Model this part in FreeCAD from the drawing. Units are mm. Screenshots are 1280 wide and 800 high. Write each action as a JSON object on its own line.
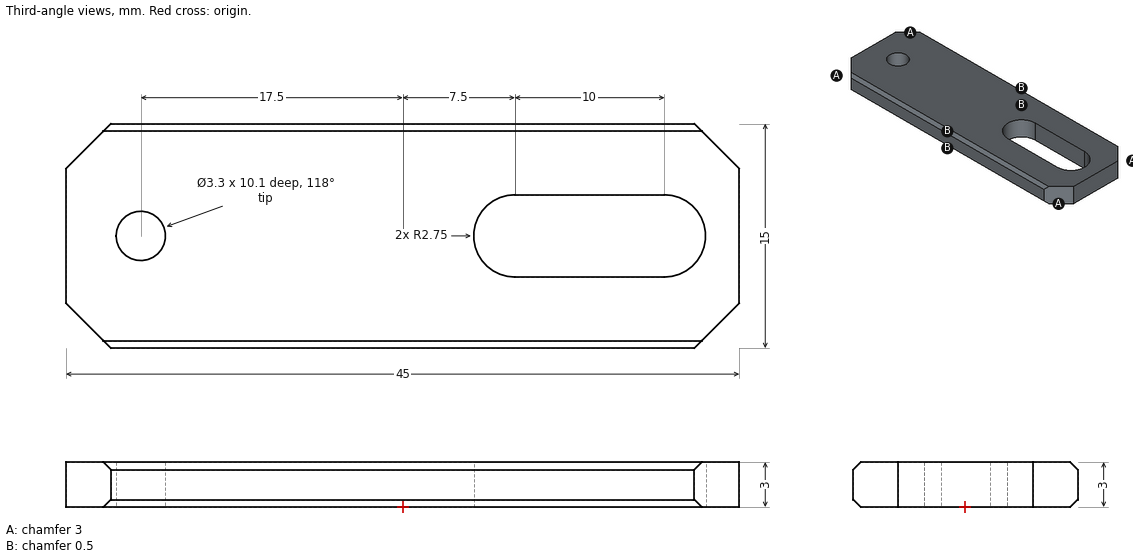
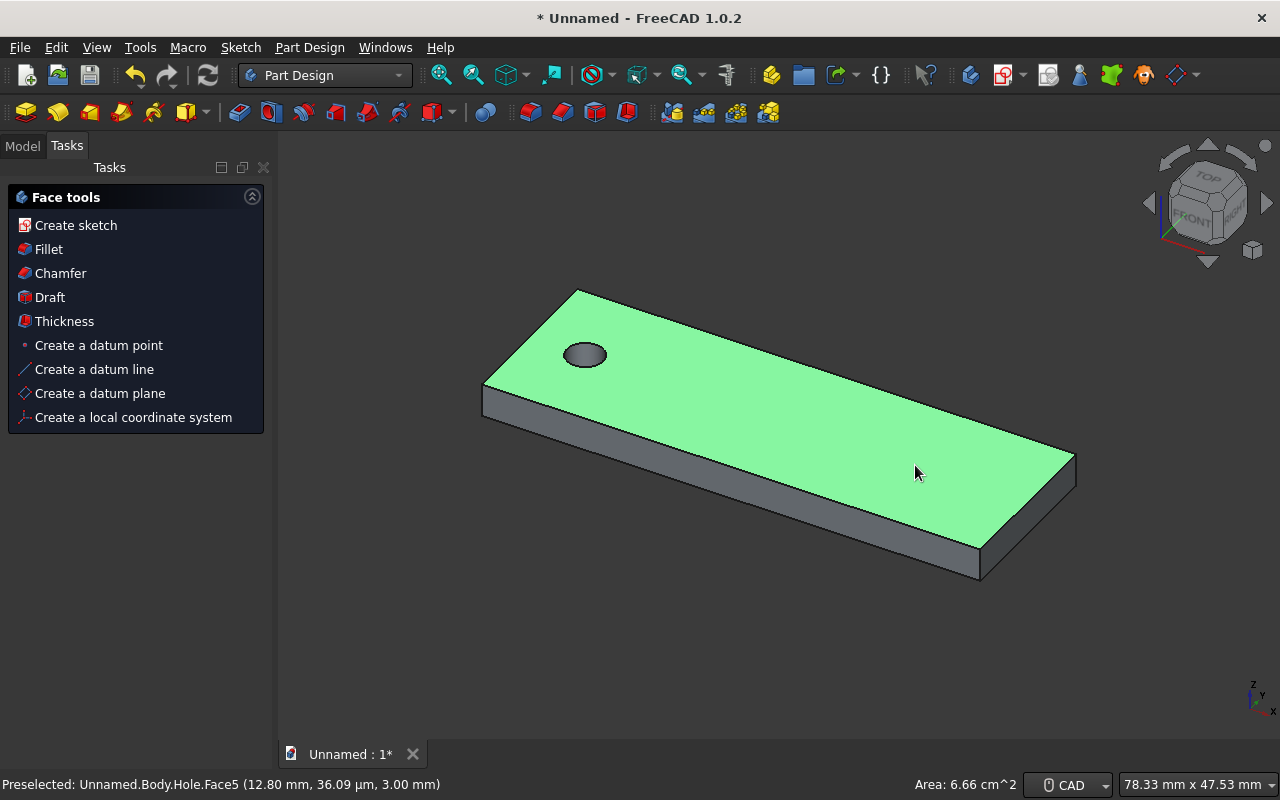
{"action": "left_click", "coordinate": [1004, 76]}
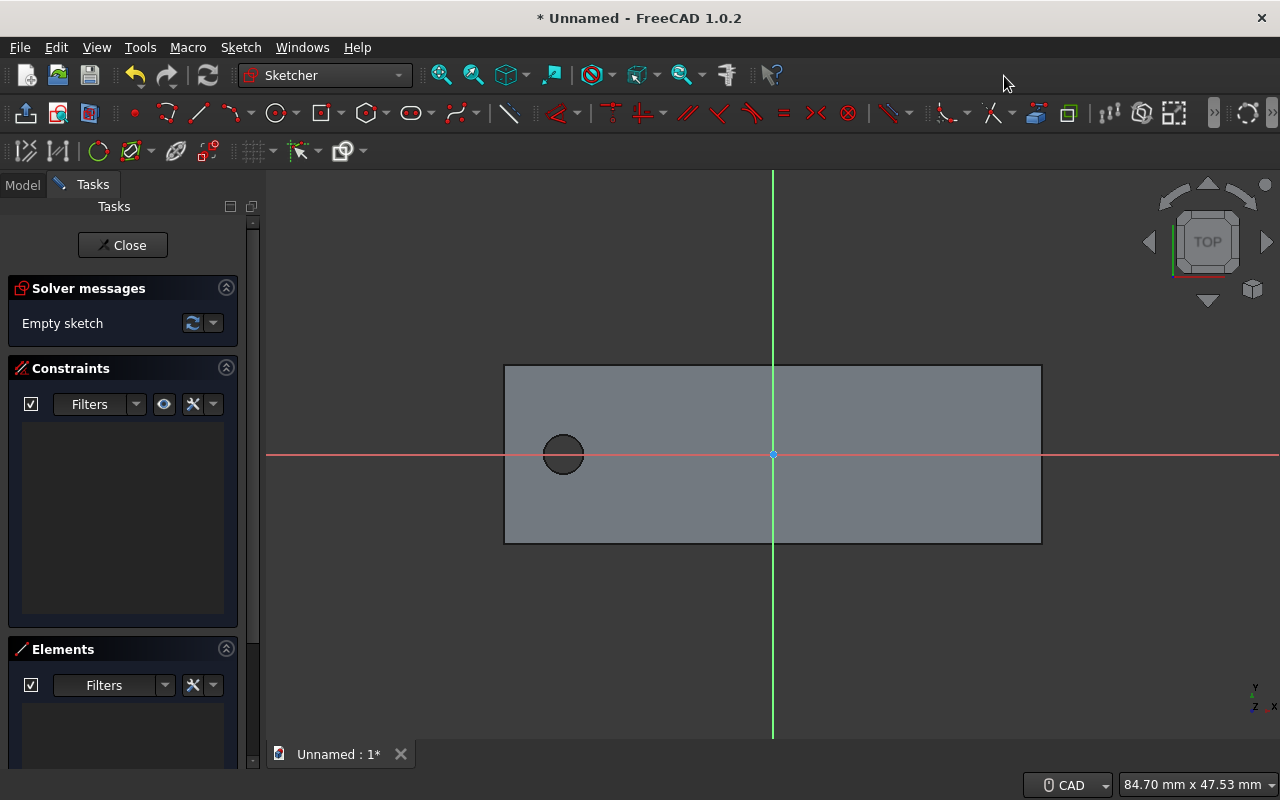
{"action": "scroll", "coordinate": [1049, 455], "scroll_direction": "up", "scroll_amount": 4}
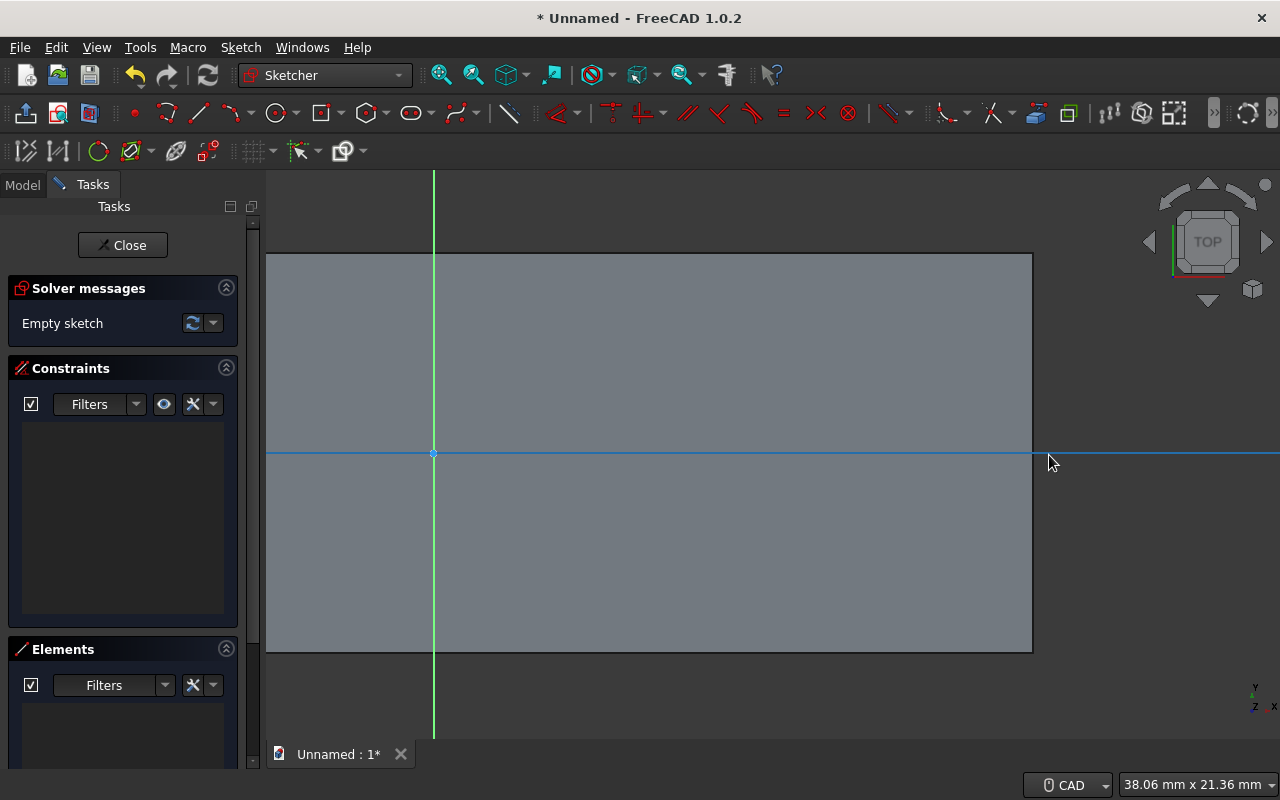
{"action": "left_click", "coordinate": [412, 114]}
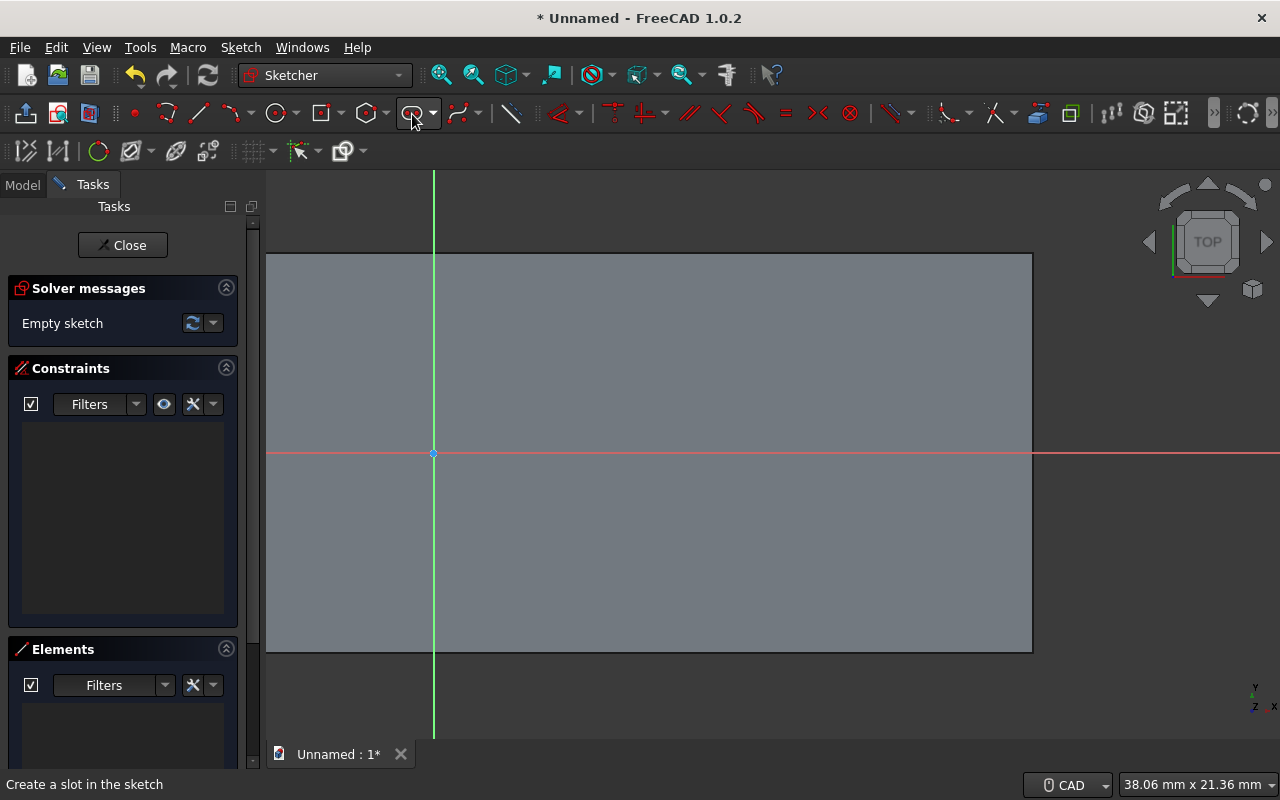
{"action": "left_click", "coordinate": [634, 453]}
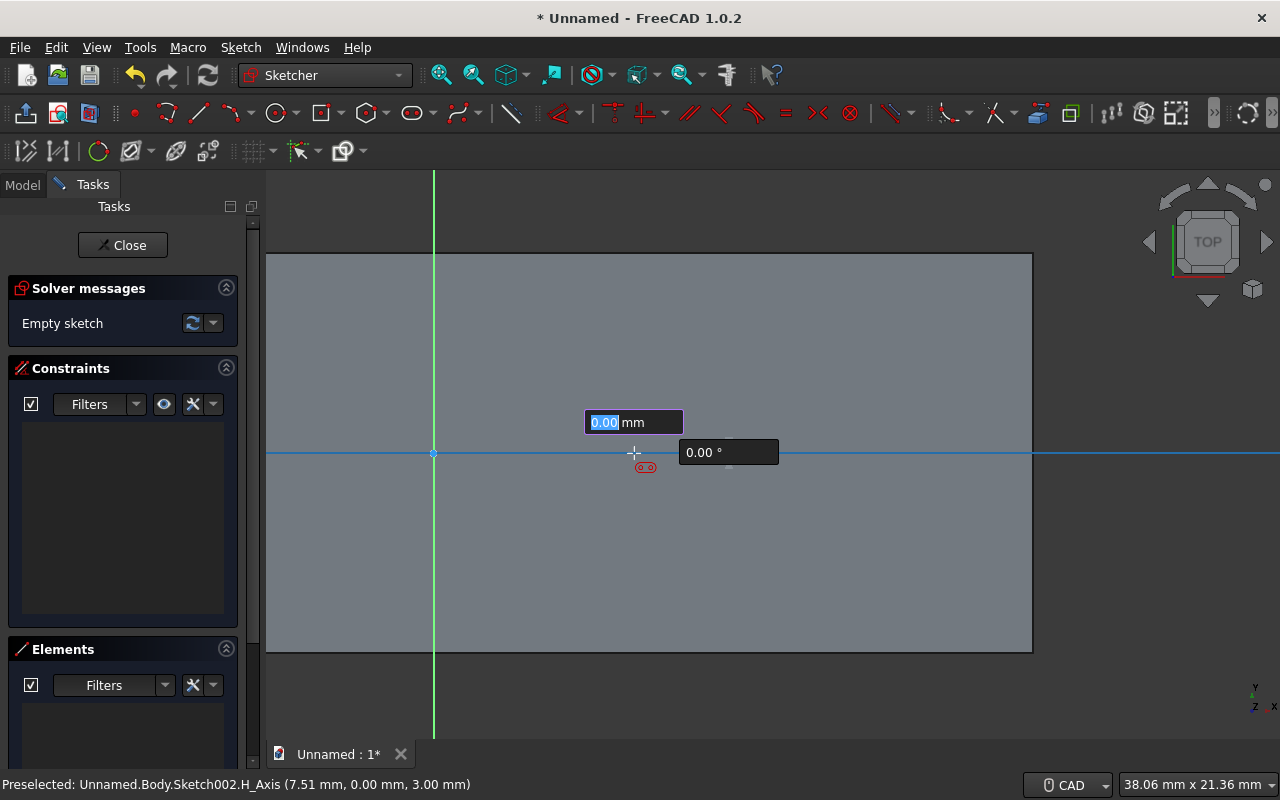
{"action": "left_click", "coordinate": [900, 444]}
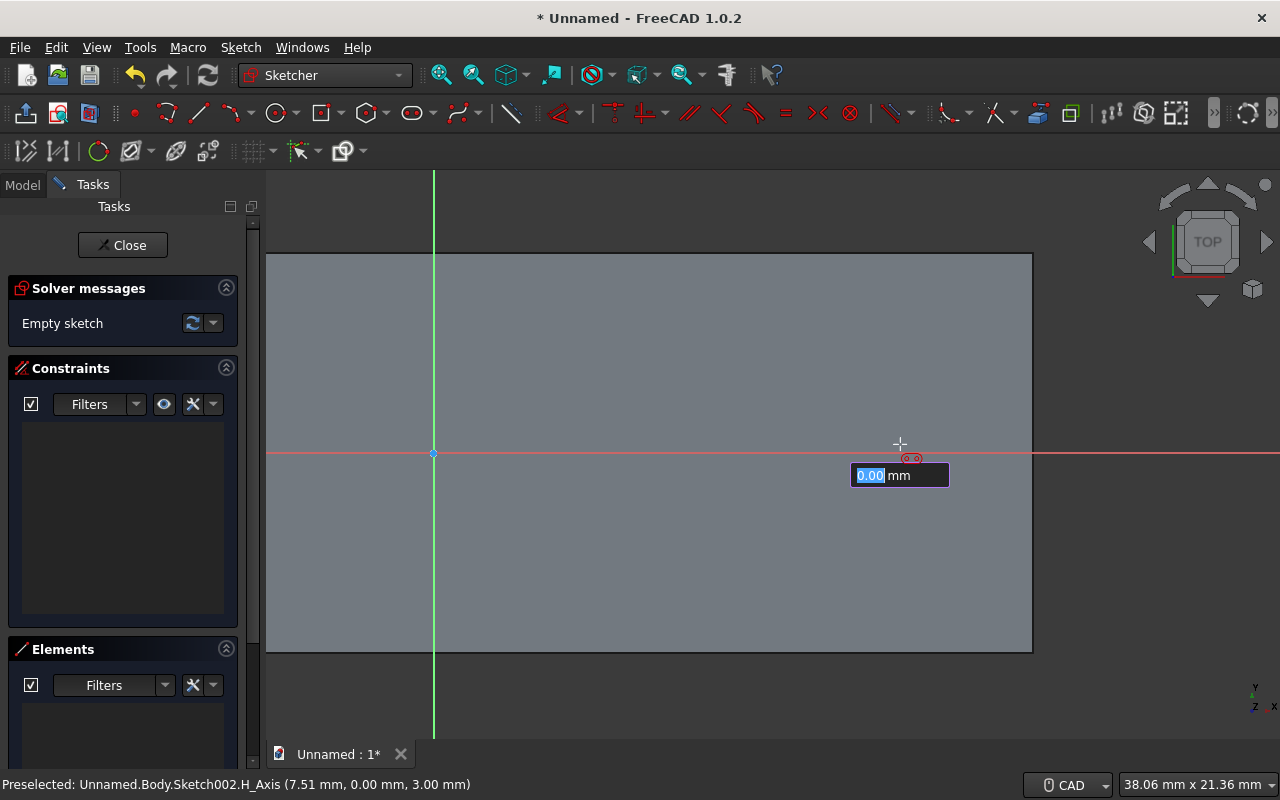
{"action": "left_click", "coordinate": [767, 380]}
{"action": "key", "text": "Escape"}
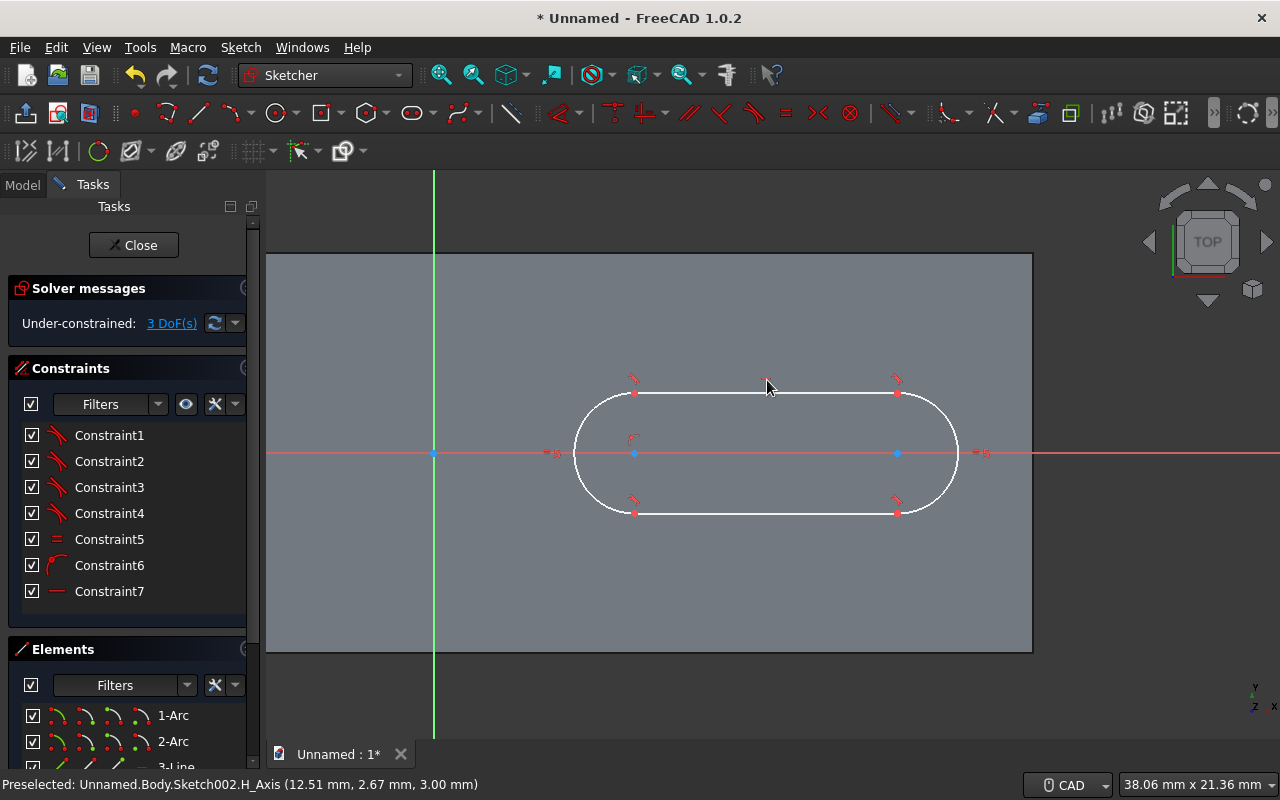
{"action": "left_click", "coordinate": [586, 418]}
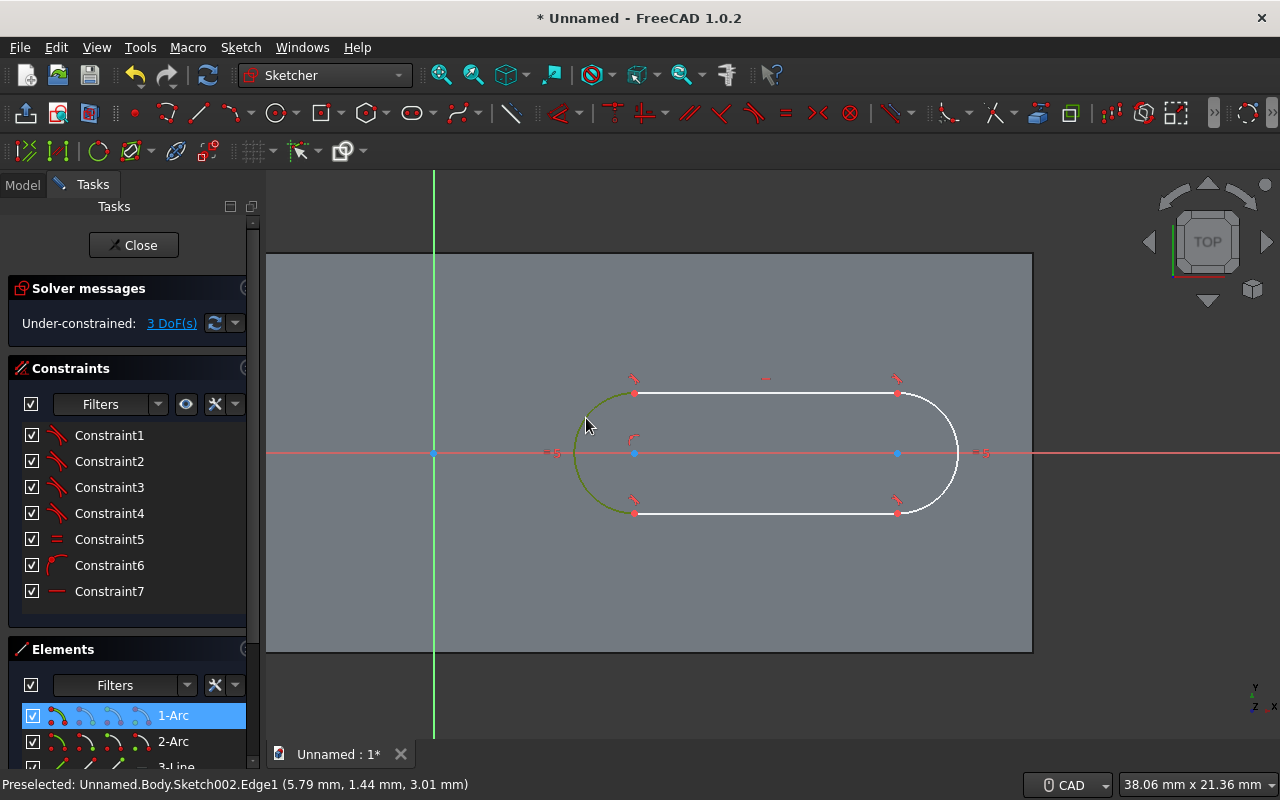
{"action": "left_click", "coordinate": [582, 114]}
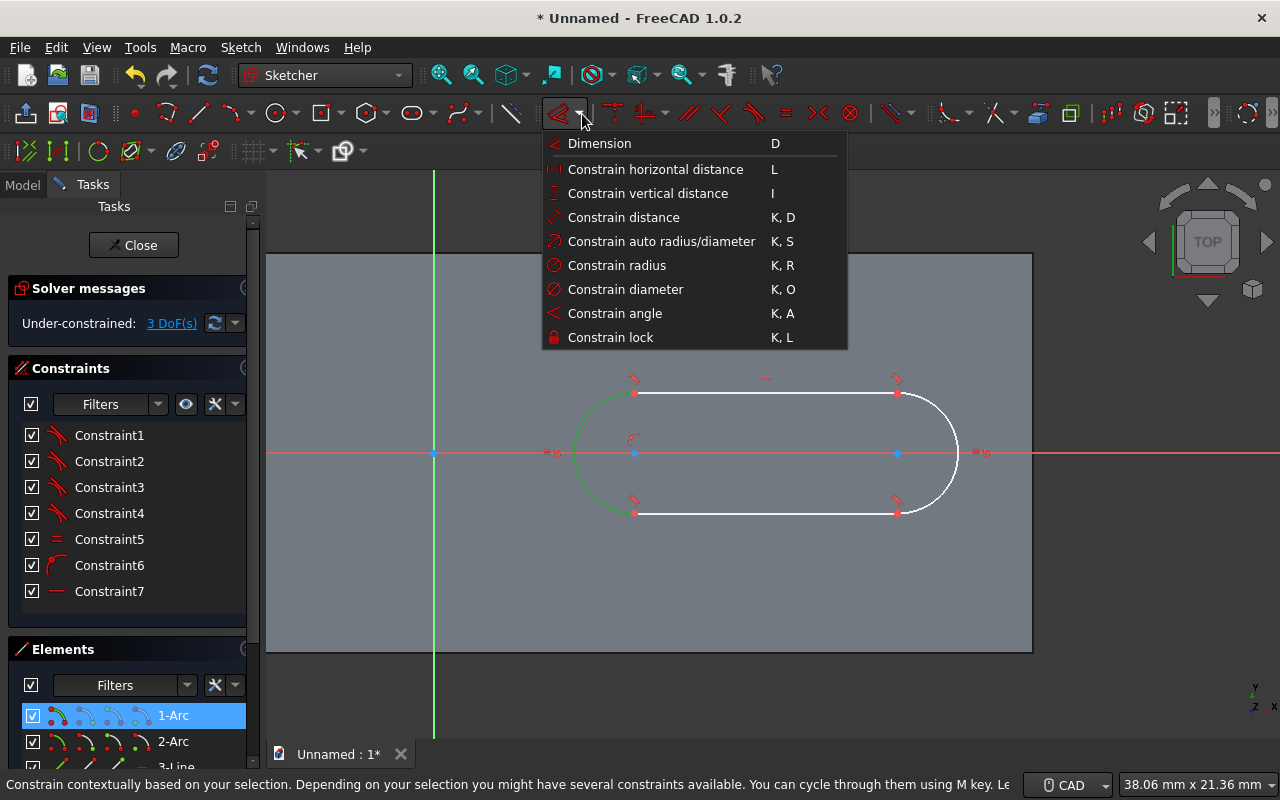
{"action": "left_click", "coordinate": [695, 265]}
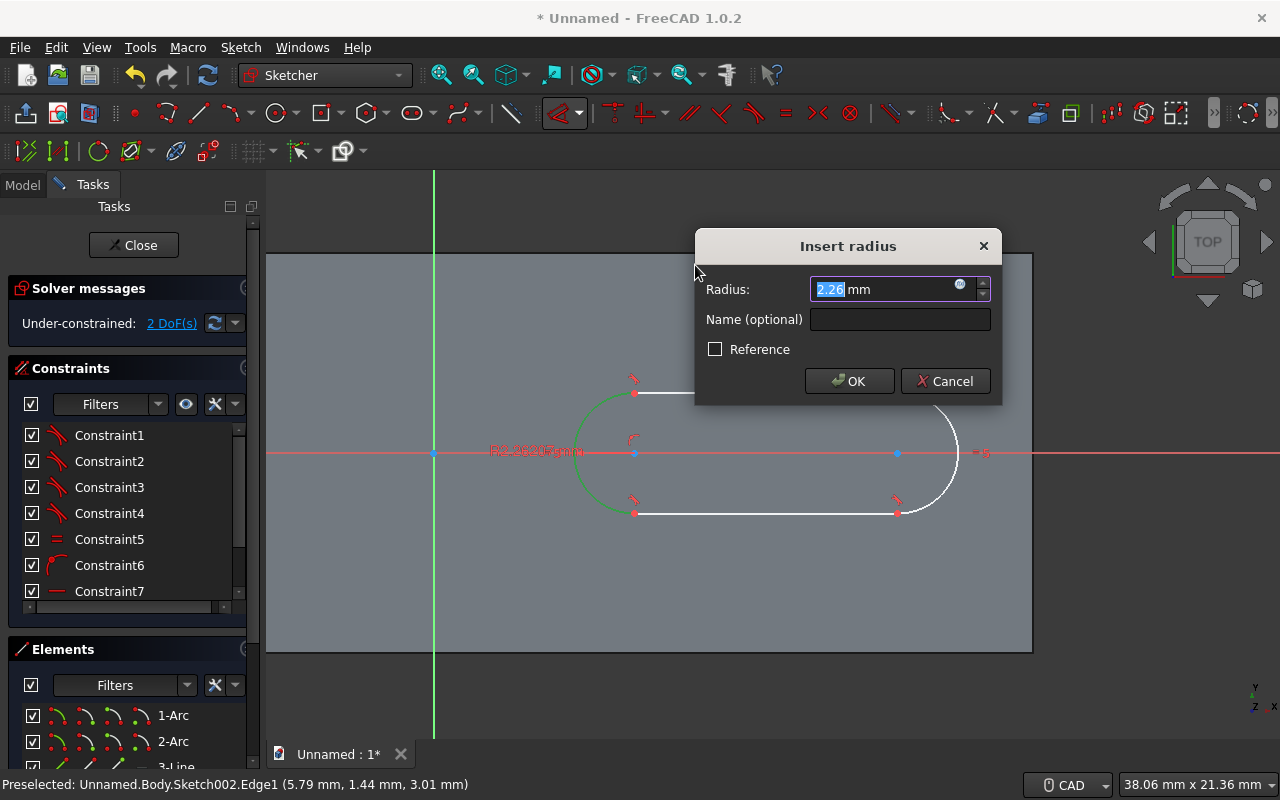
{"action": "type", "text": "2.75"}
{"action": "key", "text": "Return"}